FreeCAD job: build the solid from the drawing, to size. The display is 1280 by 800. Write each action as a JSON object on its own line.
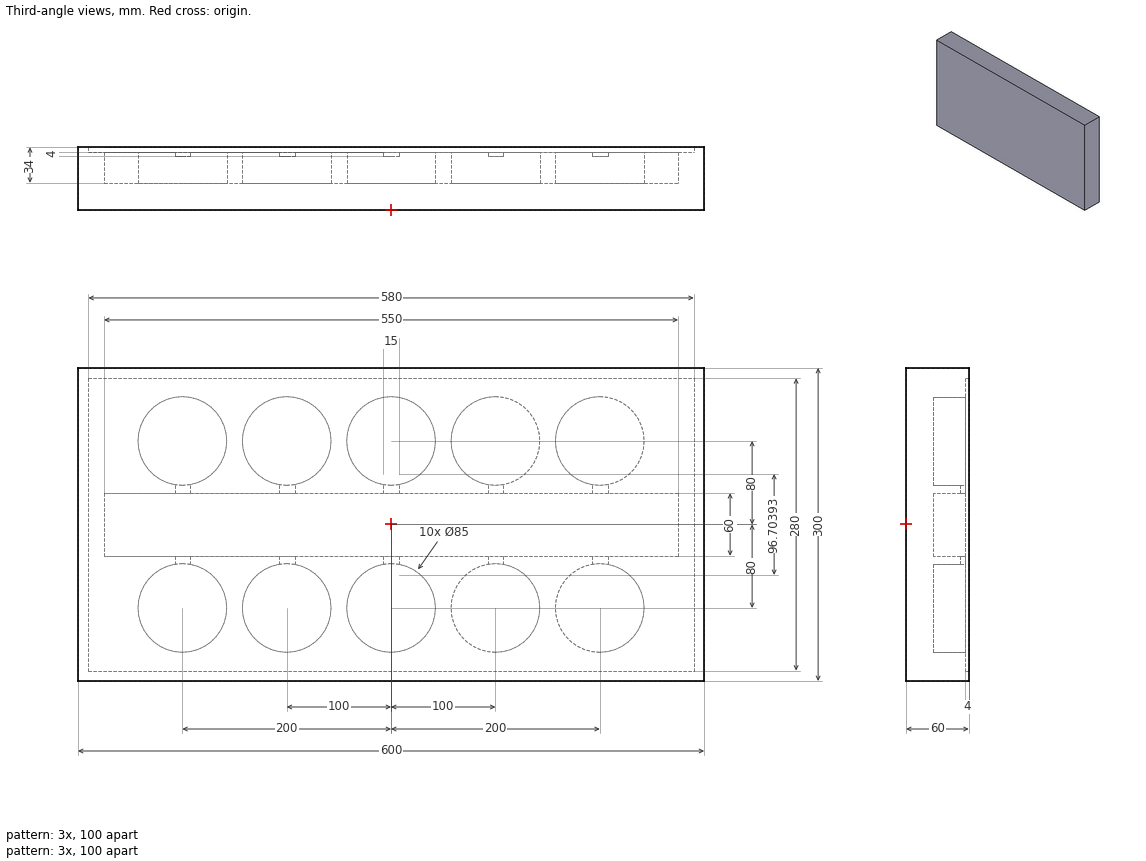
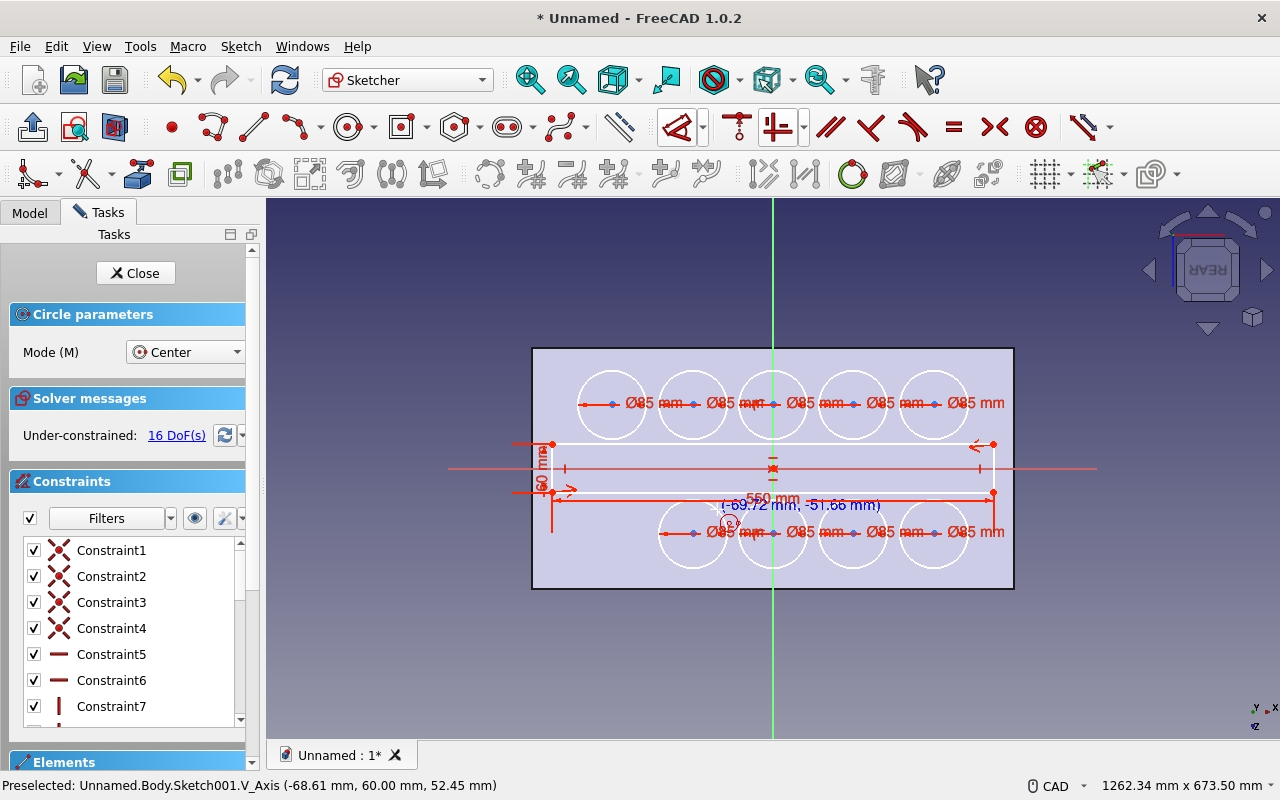
{"action": "left_click", "coordinate": [612, 533]}
{"action": "mouse_move", "coordinate": [636, 509]}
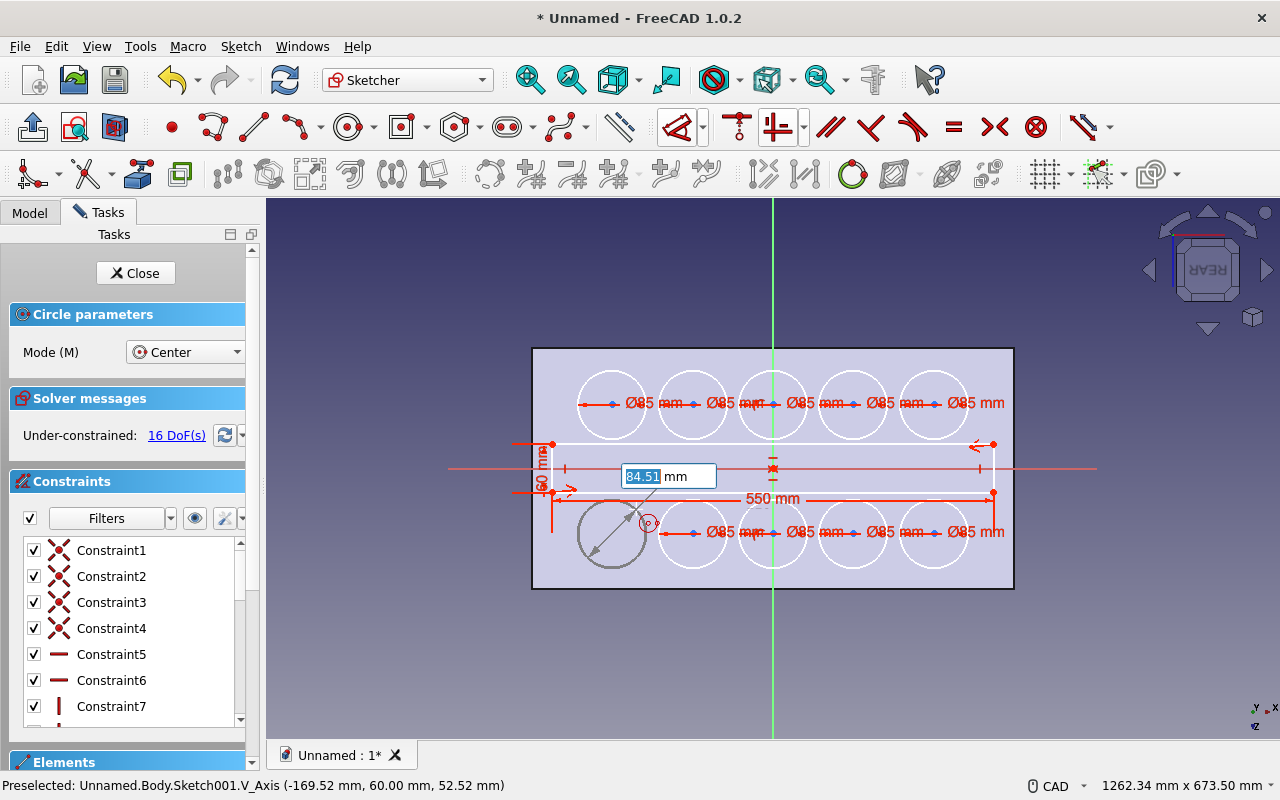
{"action": "type", "text": "85"}
{"action": "key", "text": "Return"}
{"action": "key", "text": "Escape"}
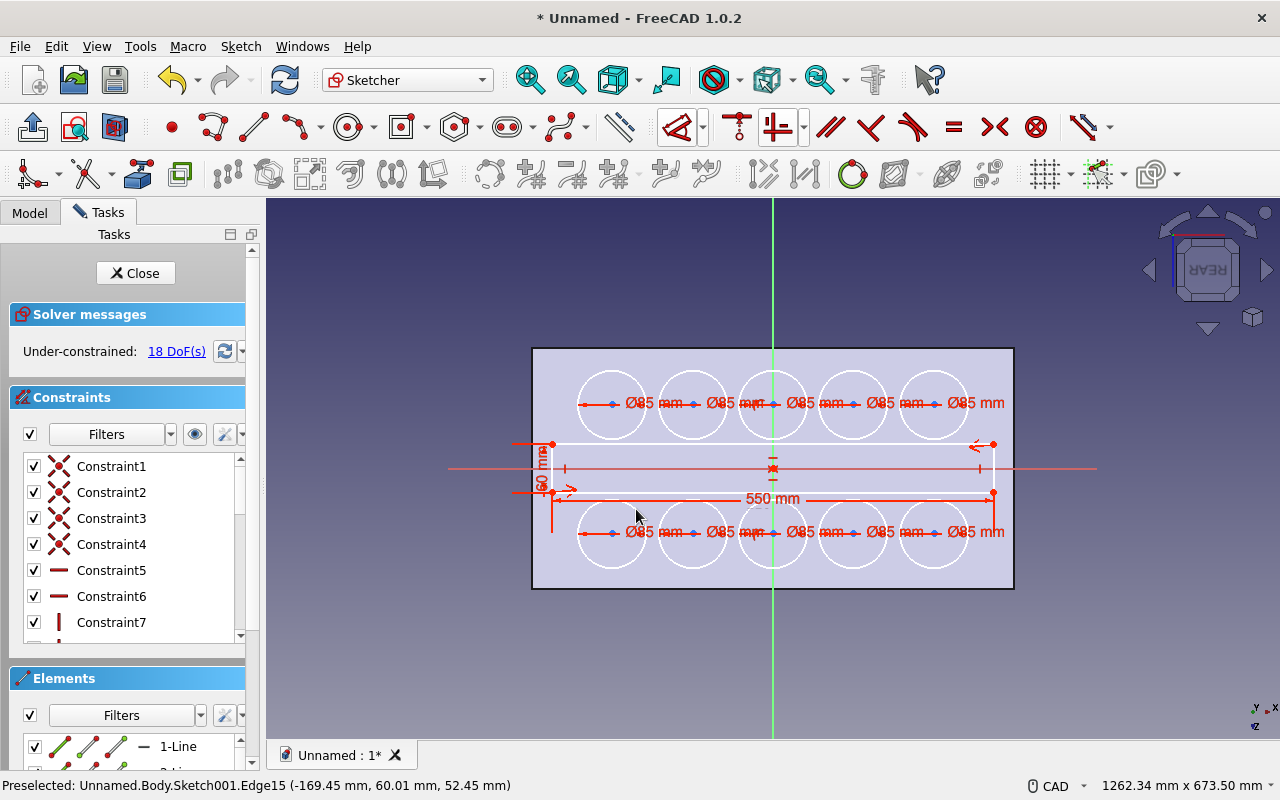
{"action": "left_click", "coordinate": [773, 405]}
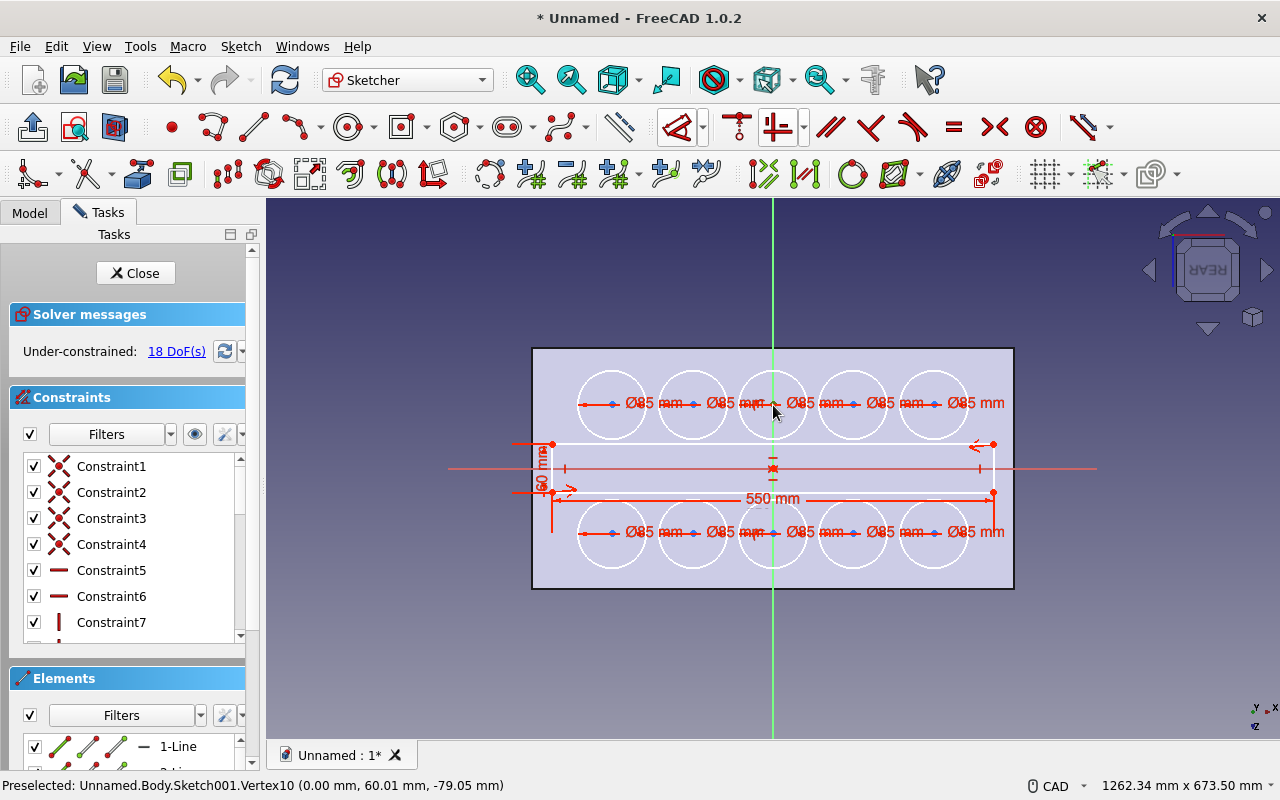
{"action": "left_click", "coordinate": [693, 405]}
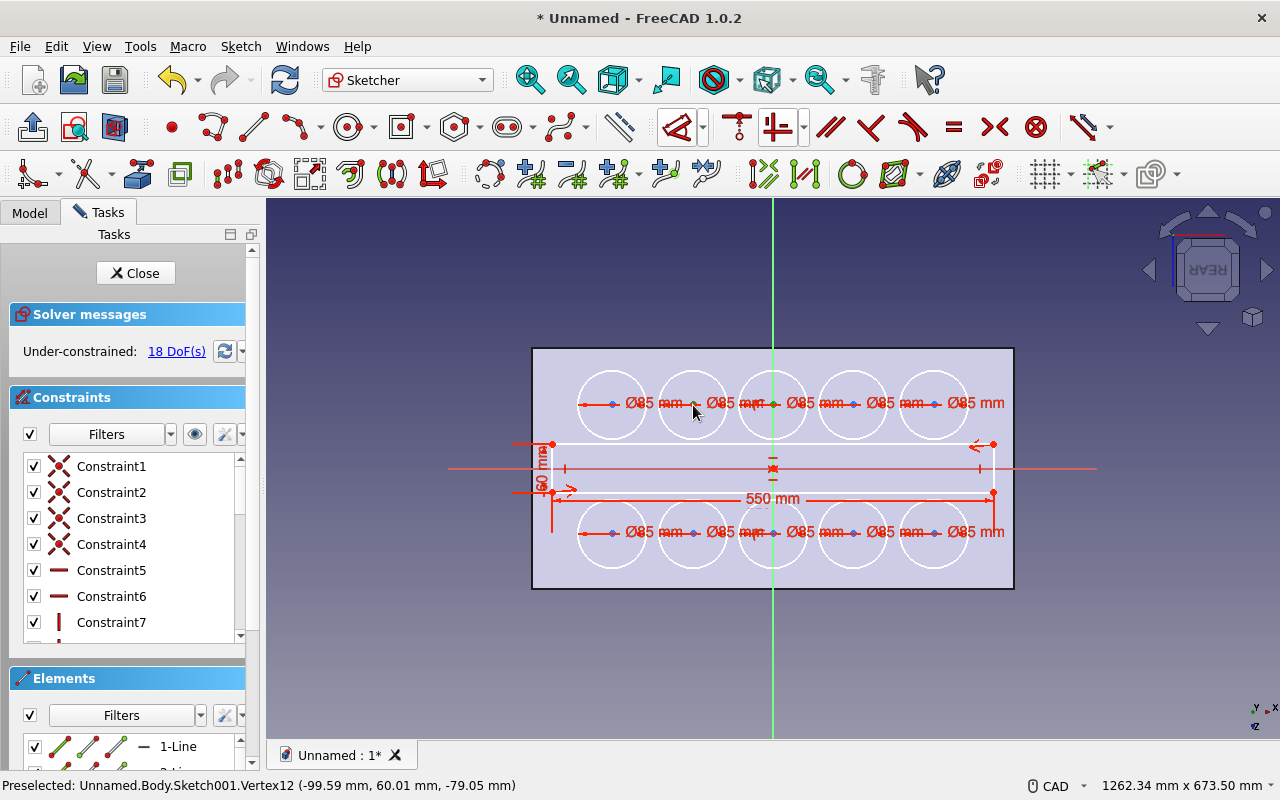
{"action": "left_click", "coordinate": [804, 128]}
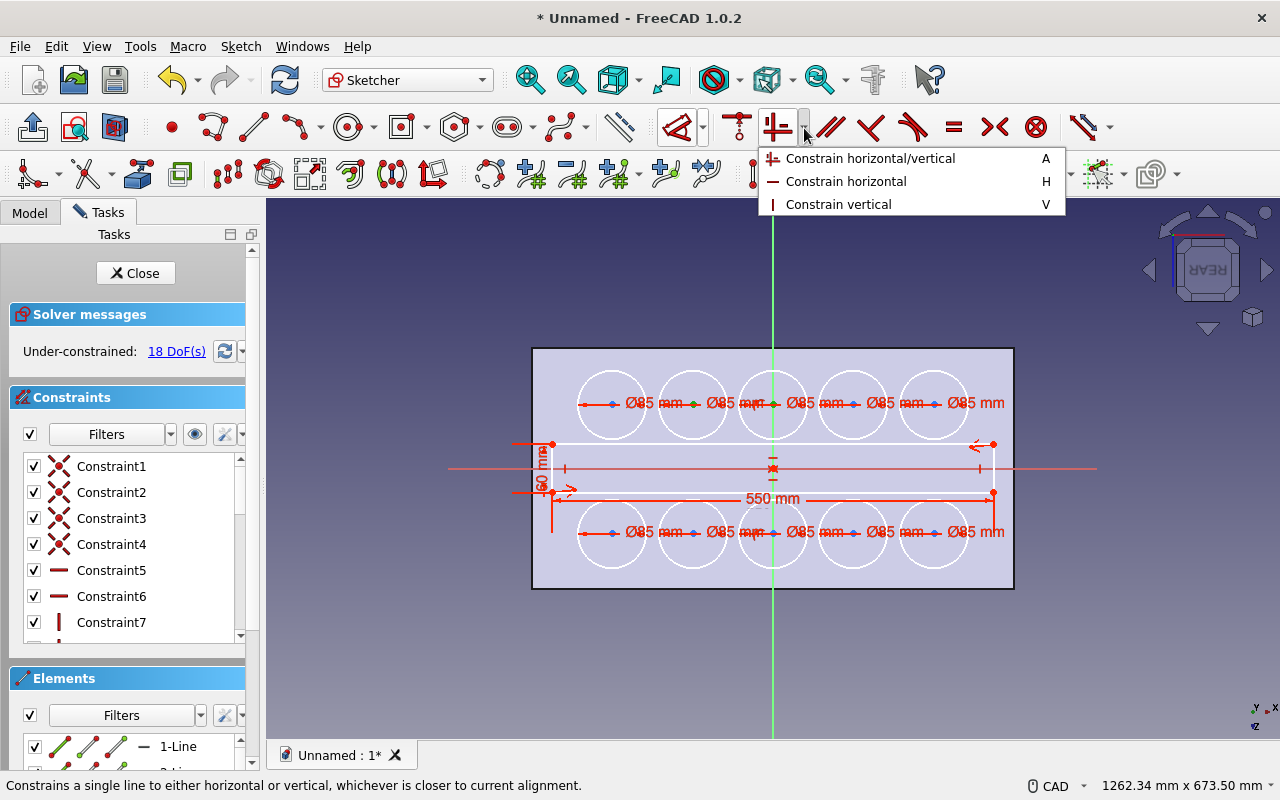
{"action": "left_click", "coordinate": [912, 182]}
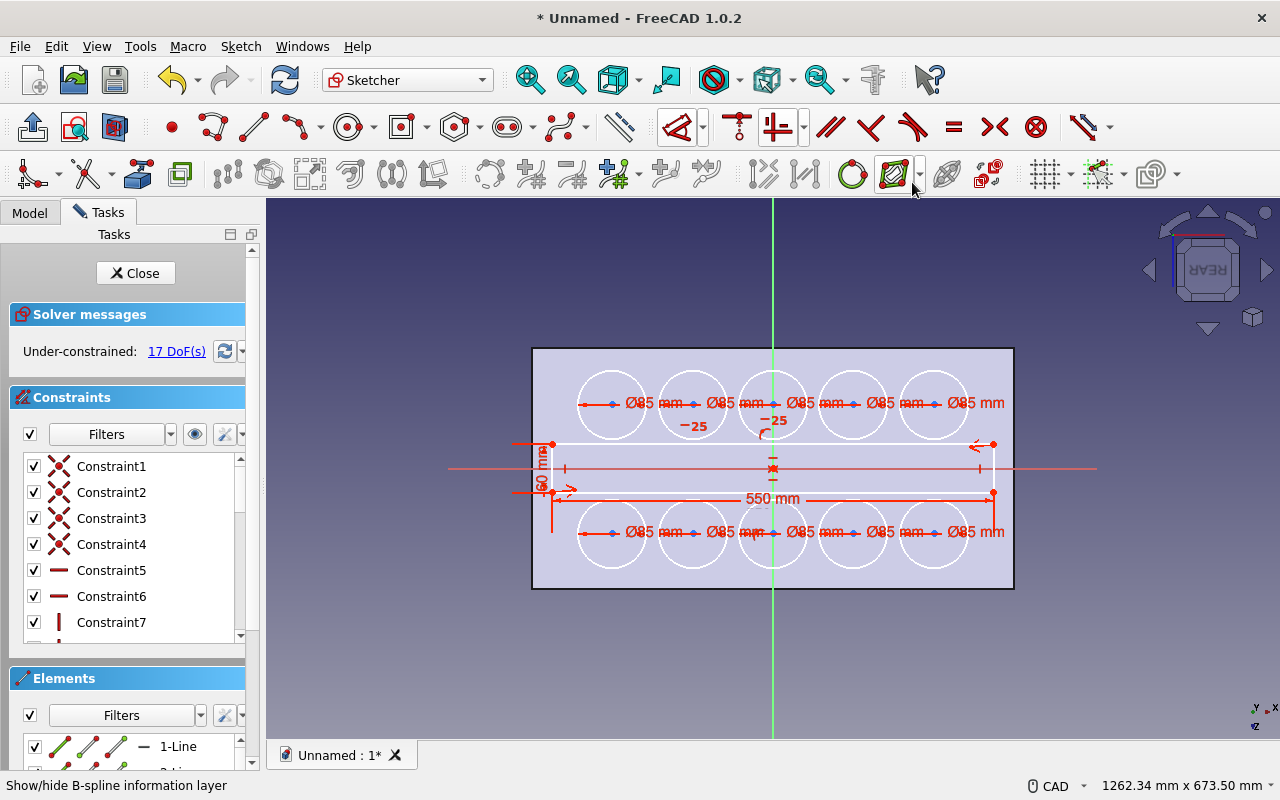
{"action": "left_click", "coordinate": [693, 405]}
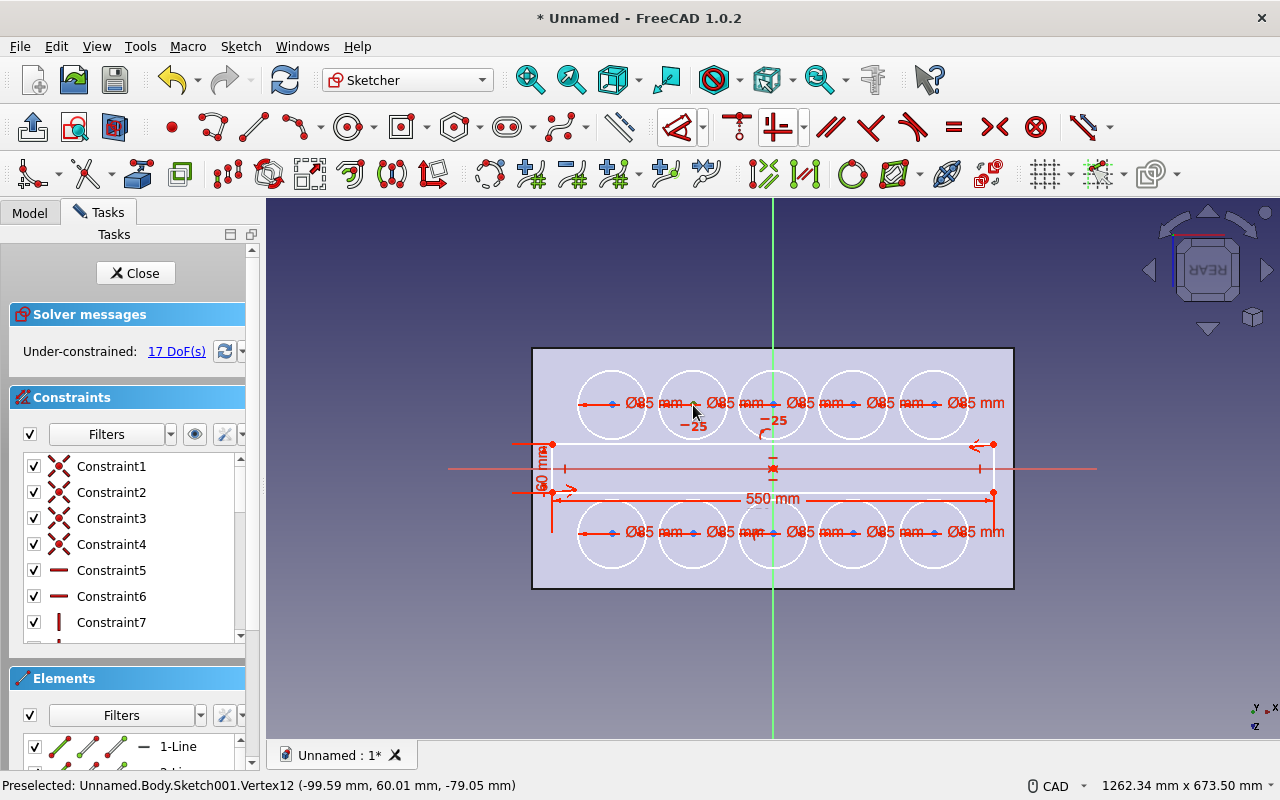
{"action": "left_click", "coordinate": [612, 405]}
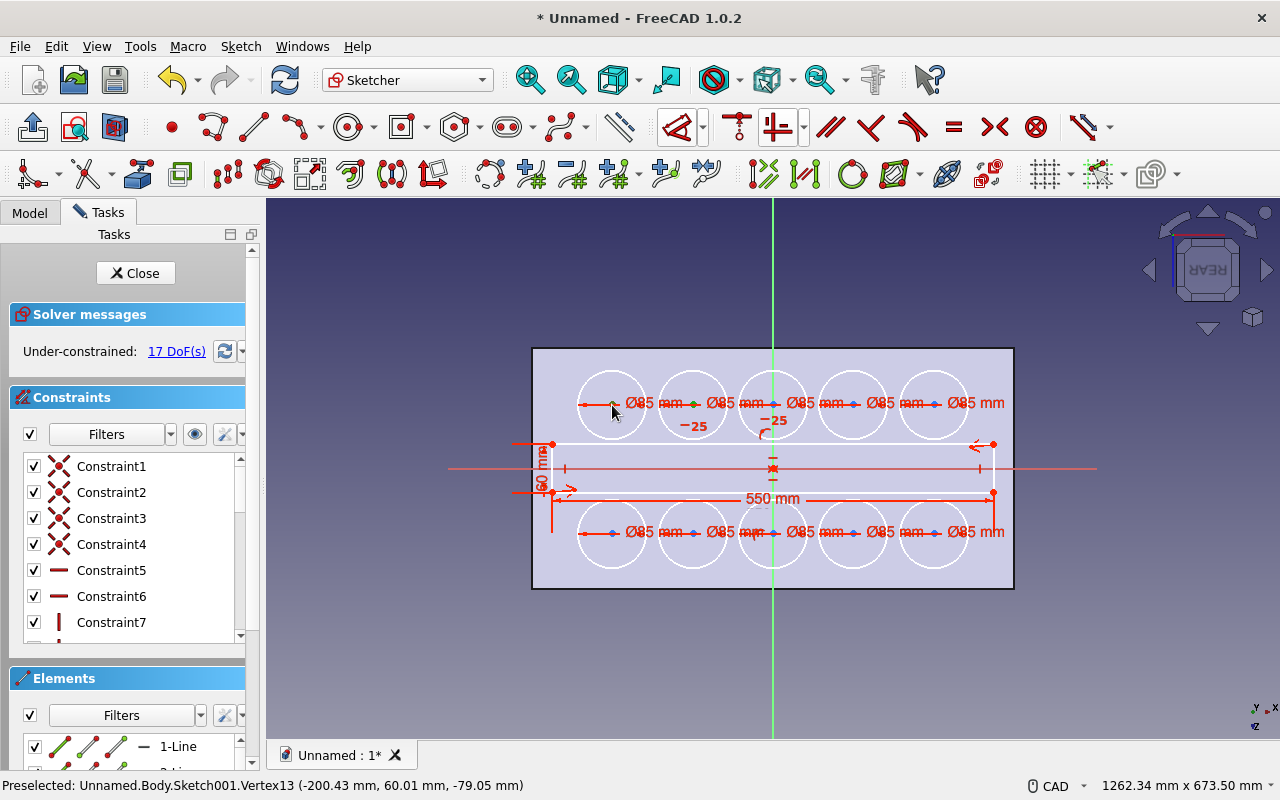
{"action": "left_click", "coordinate": [804, 128]}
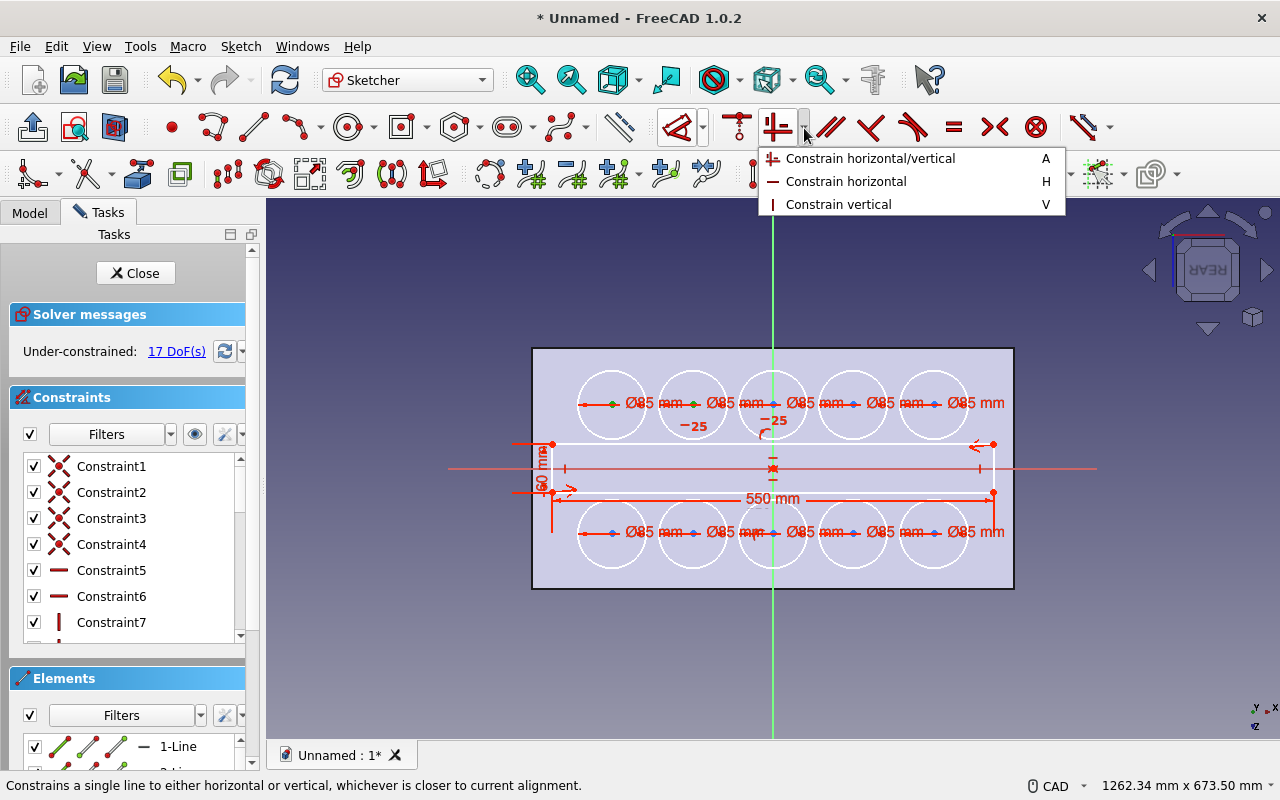
{"action": "left_click", "coordinate": [912, 182]}